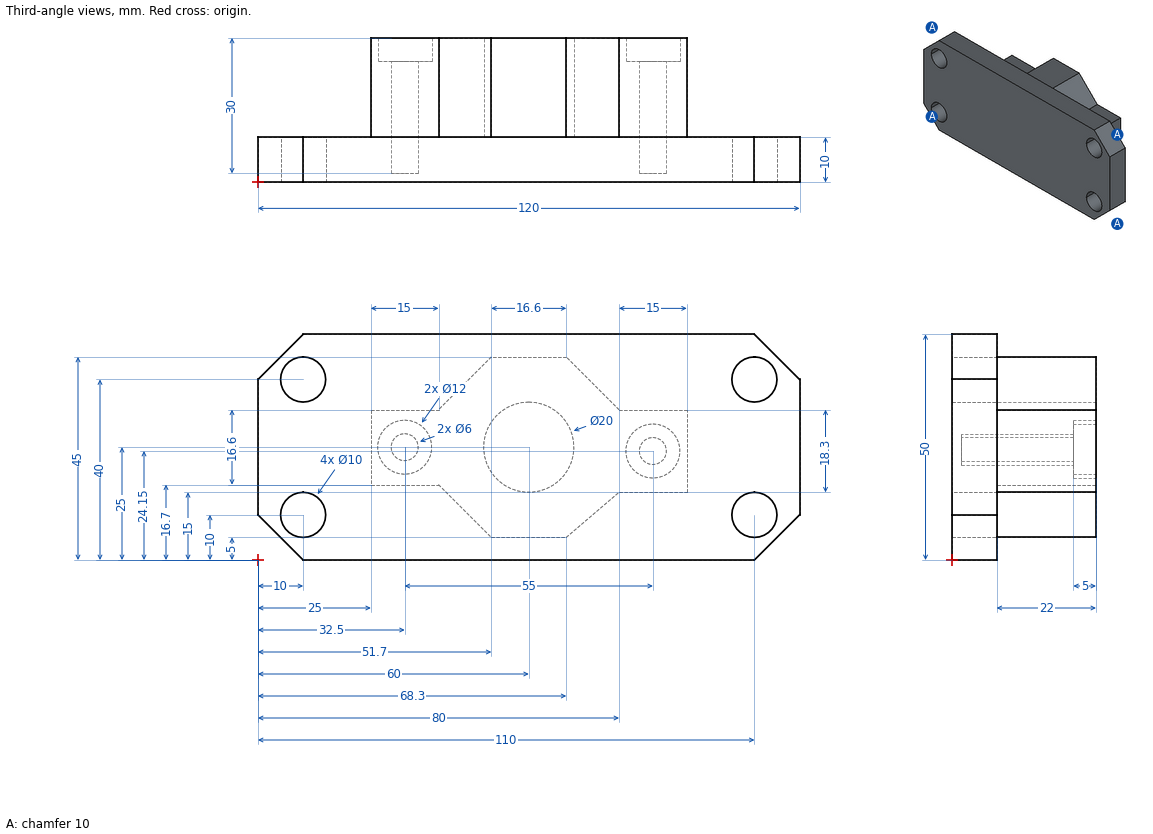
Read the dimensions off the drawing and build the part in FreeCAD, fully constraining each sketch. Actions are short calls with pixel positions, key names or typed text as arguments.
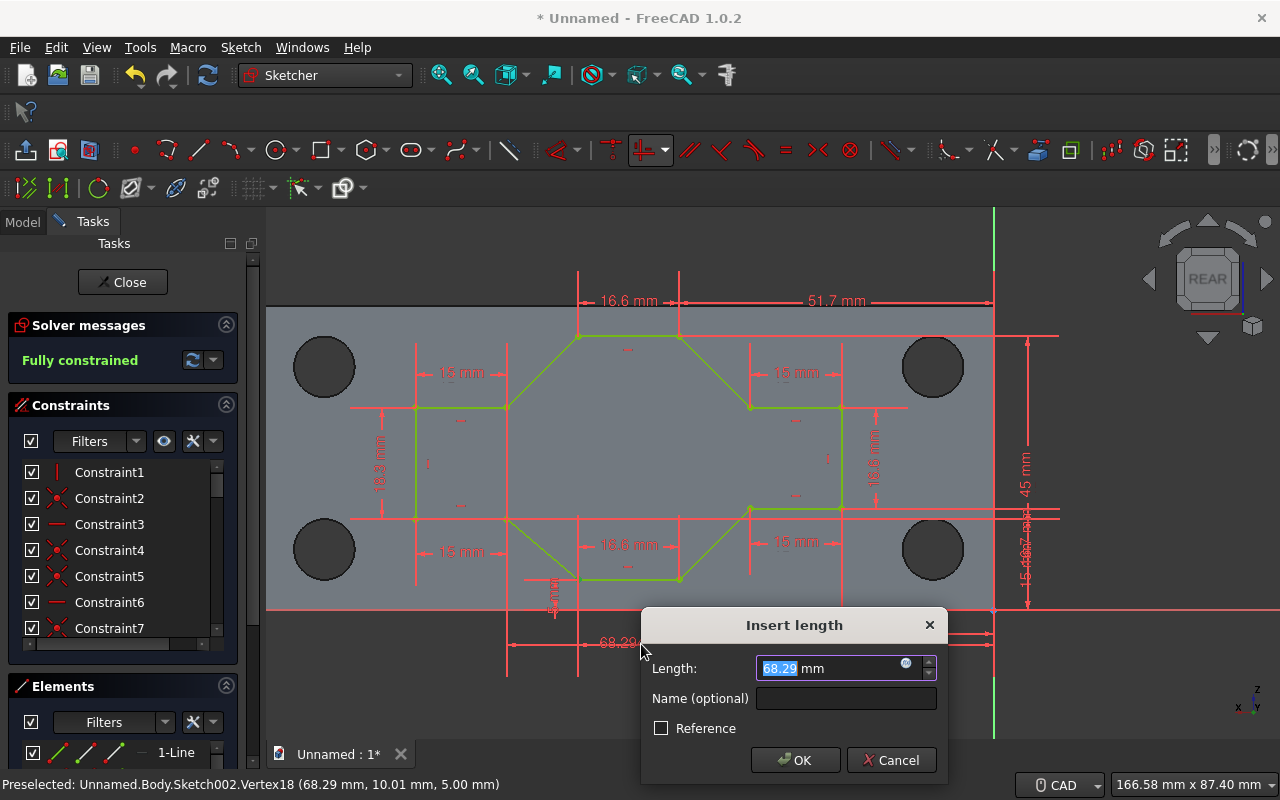
text(68.3)
key(Return)
key(Escape)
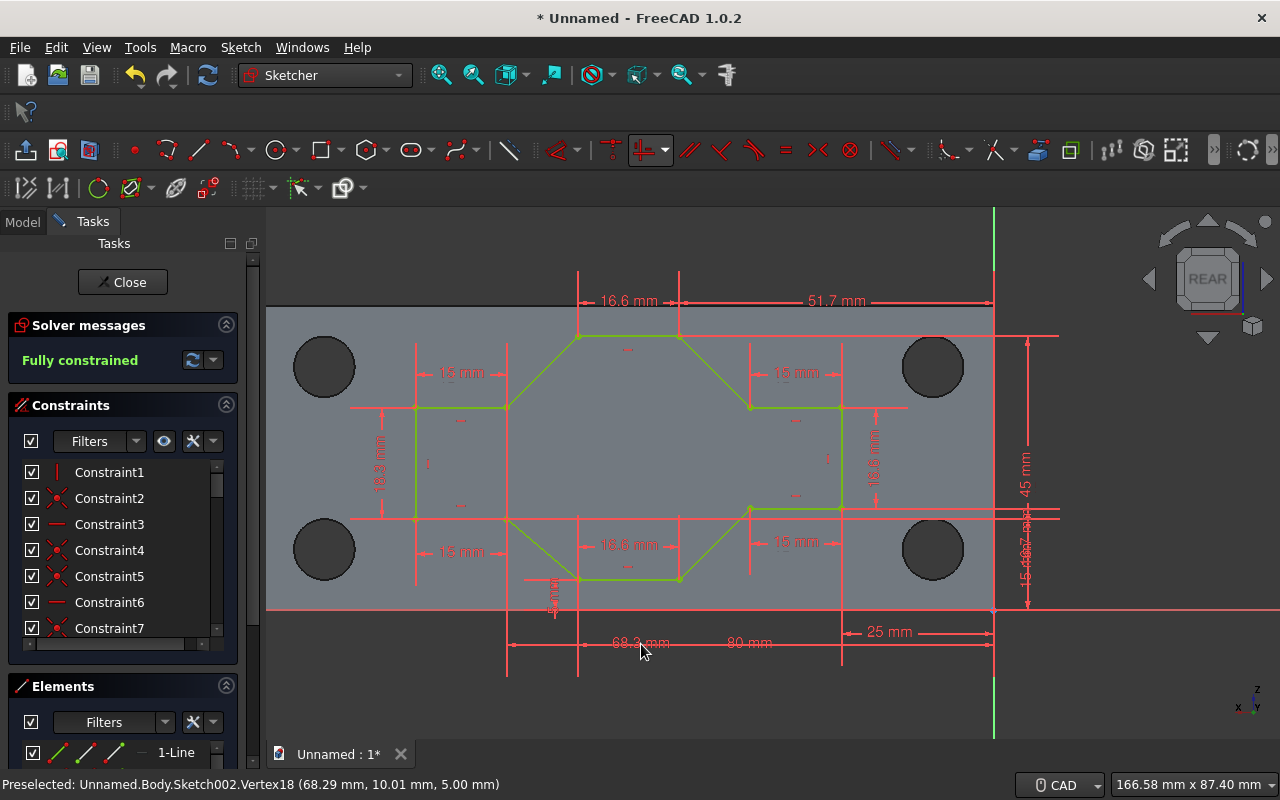
click(123, 282)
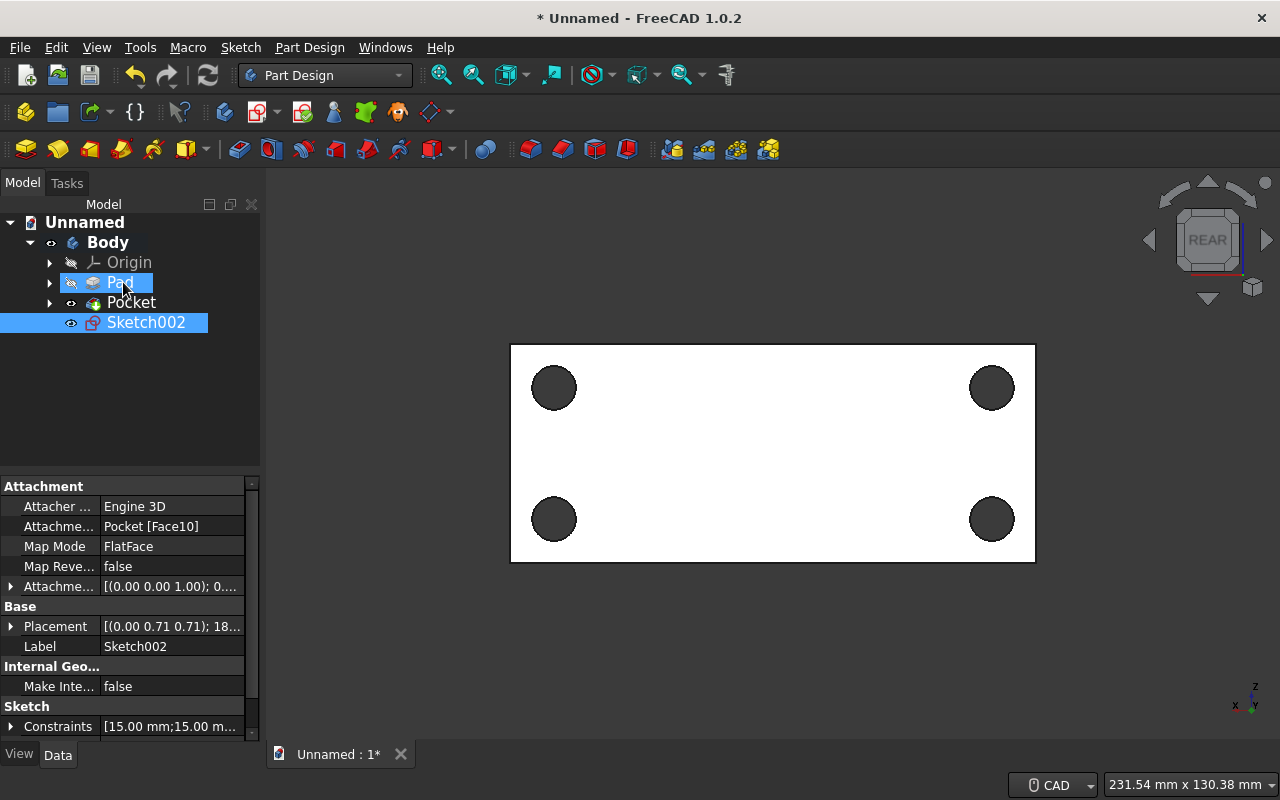
click(26, 150)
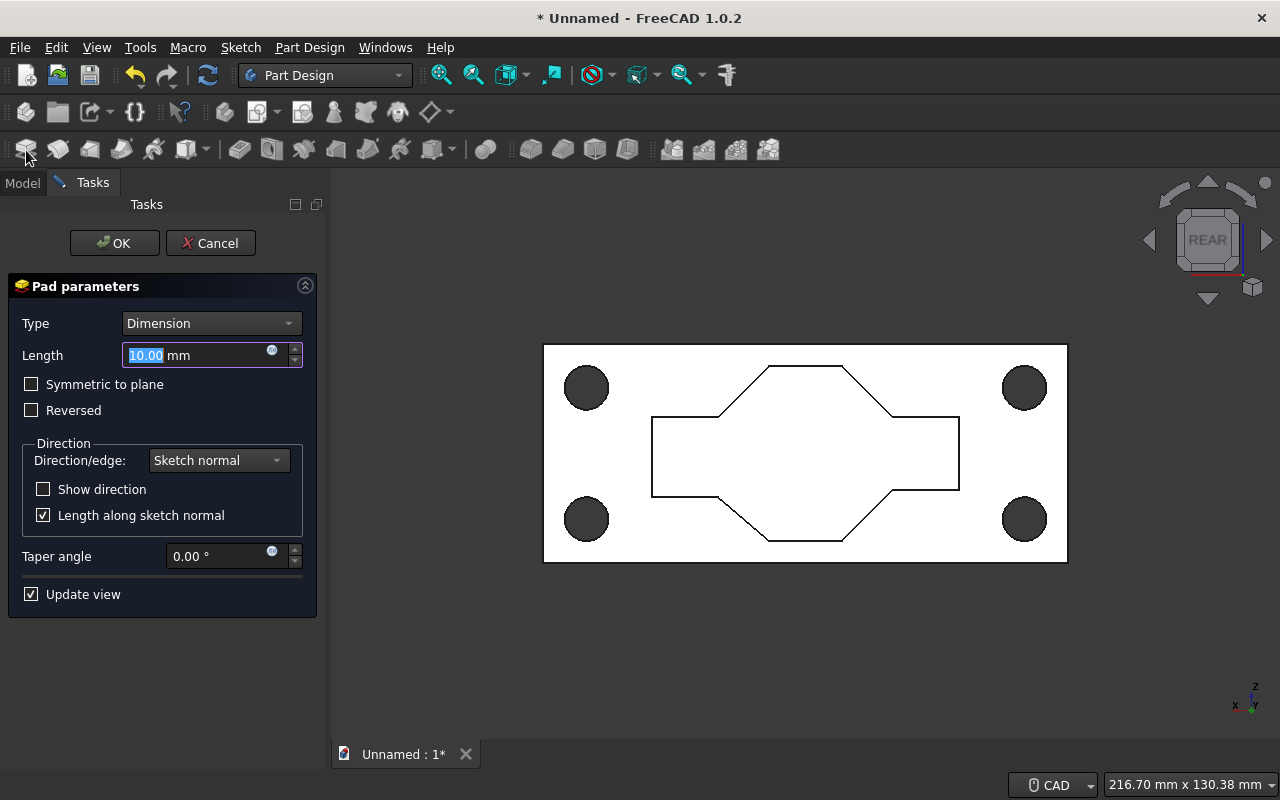
text(22)
key(Tab)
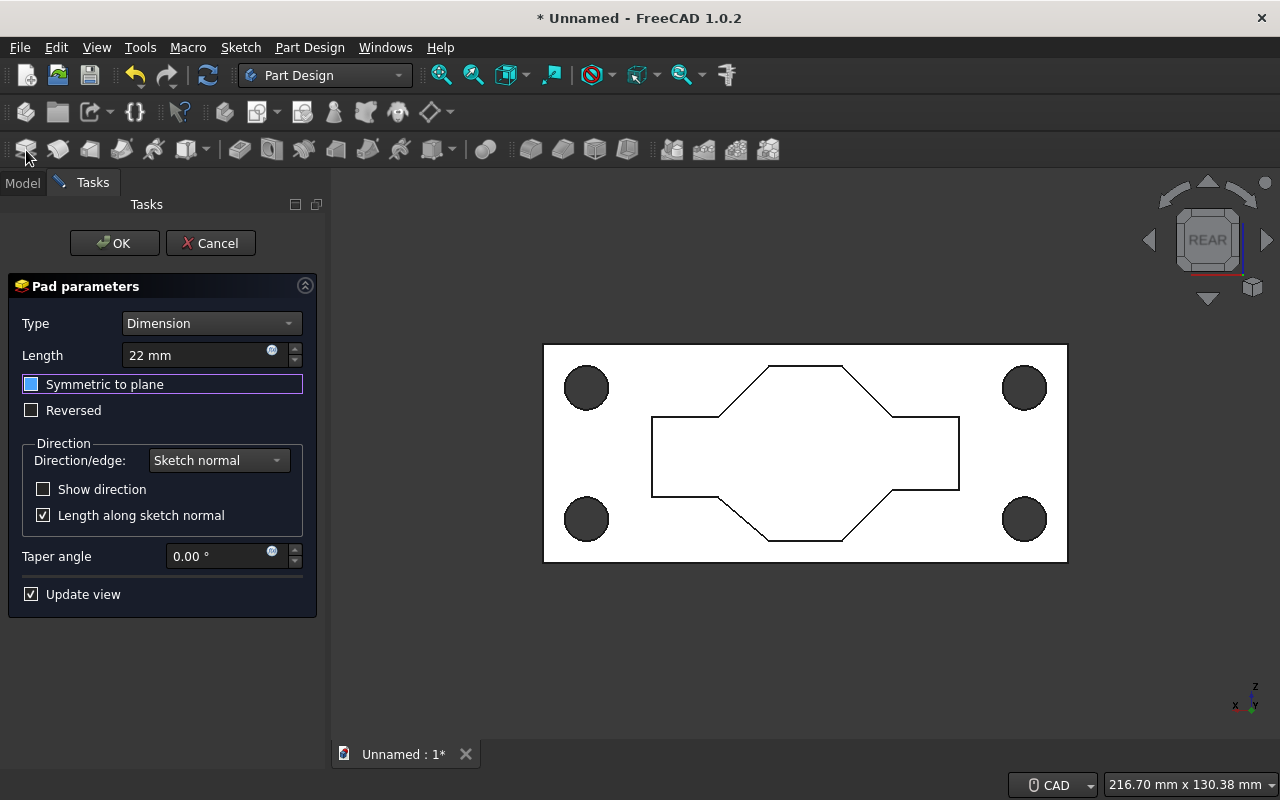
click(115, 243)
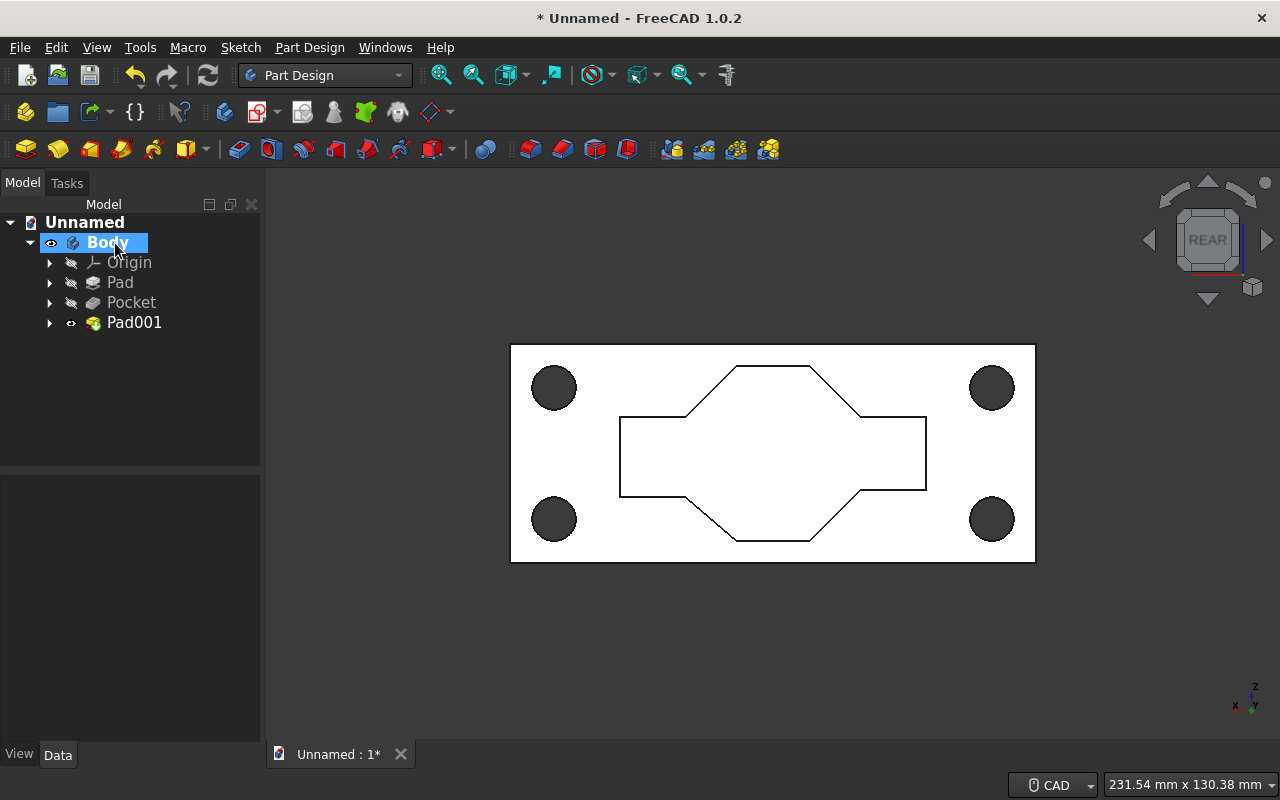
click(773, 452)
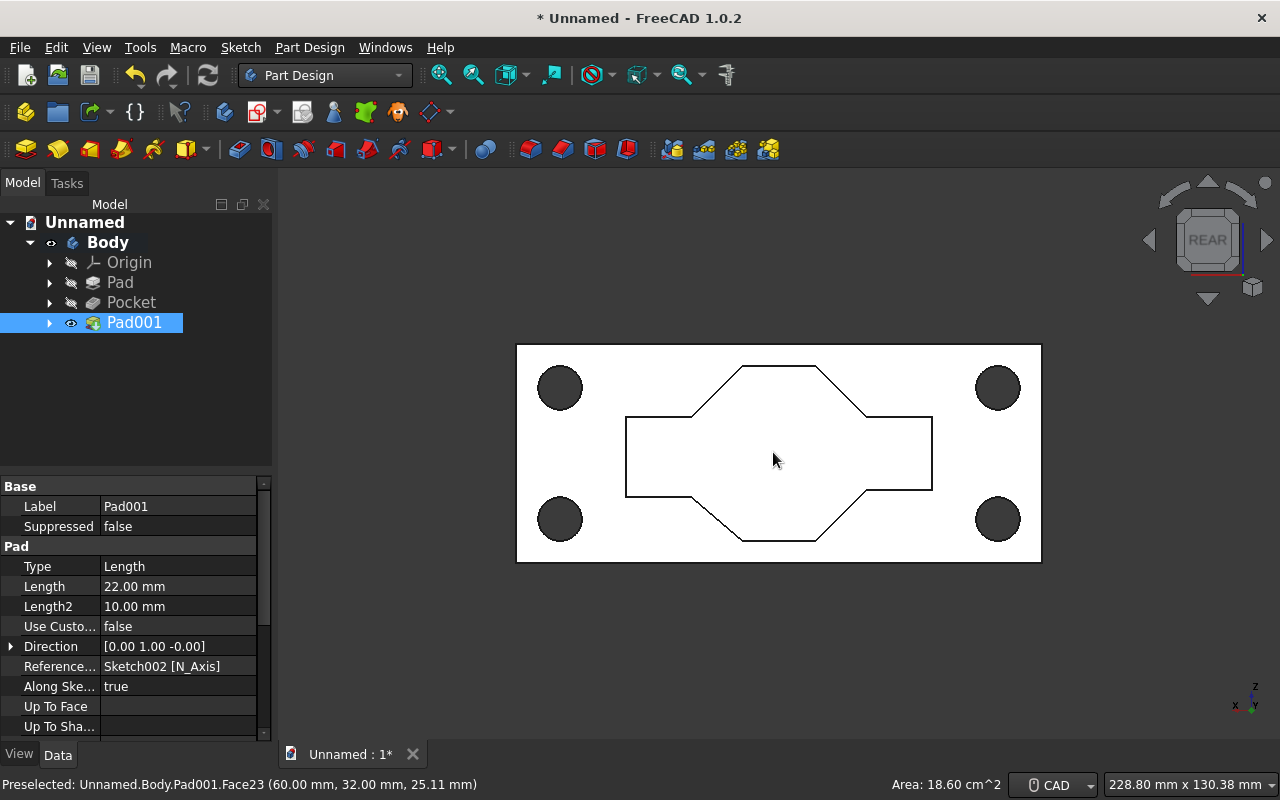
click(258, 112)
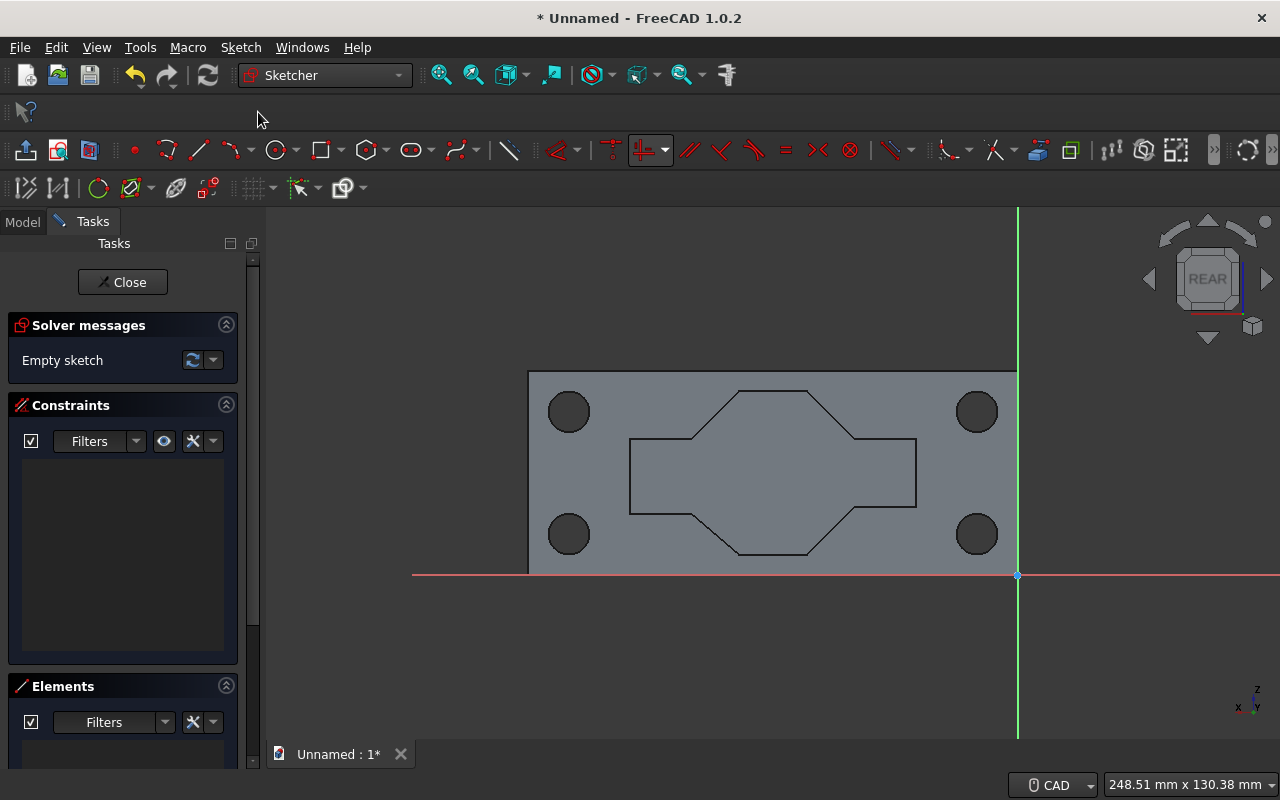
scroll(795, 473, up, 7)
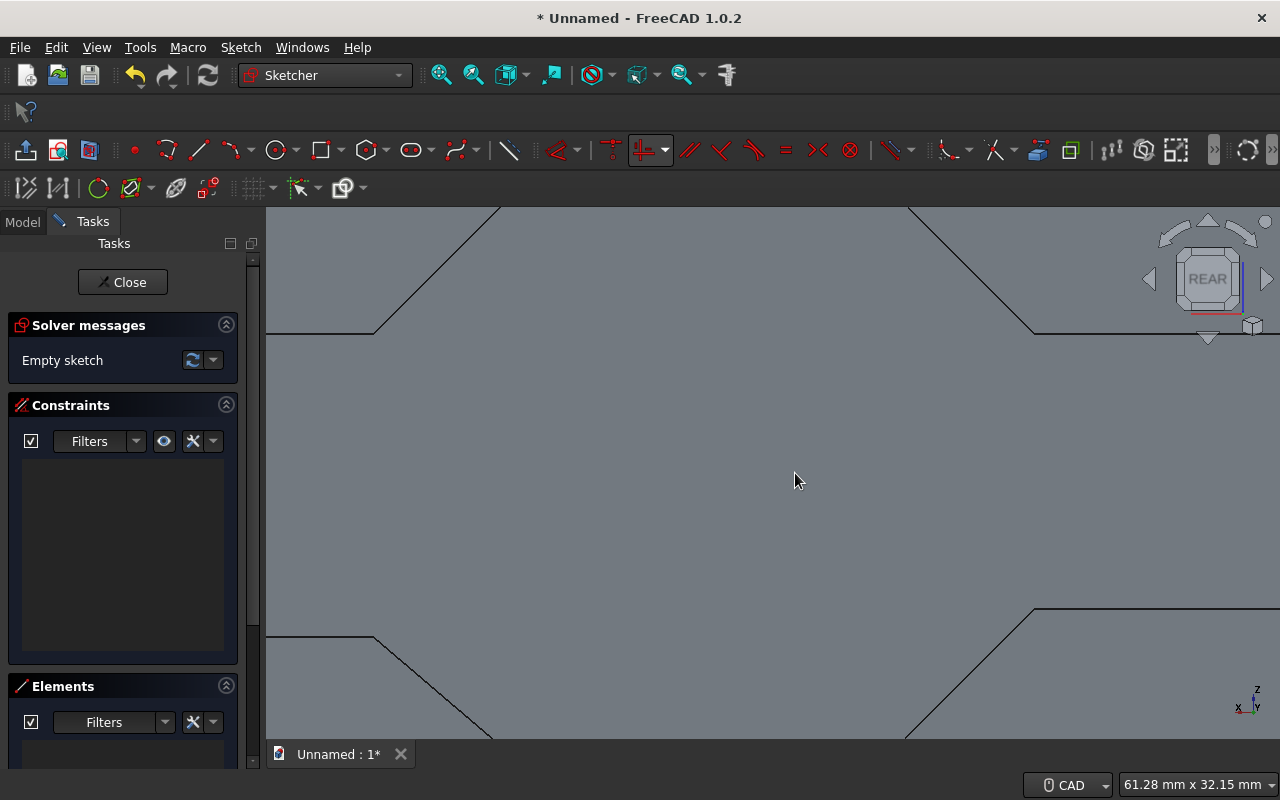
click(276, 150)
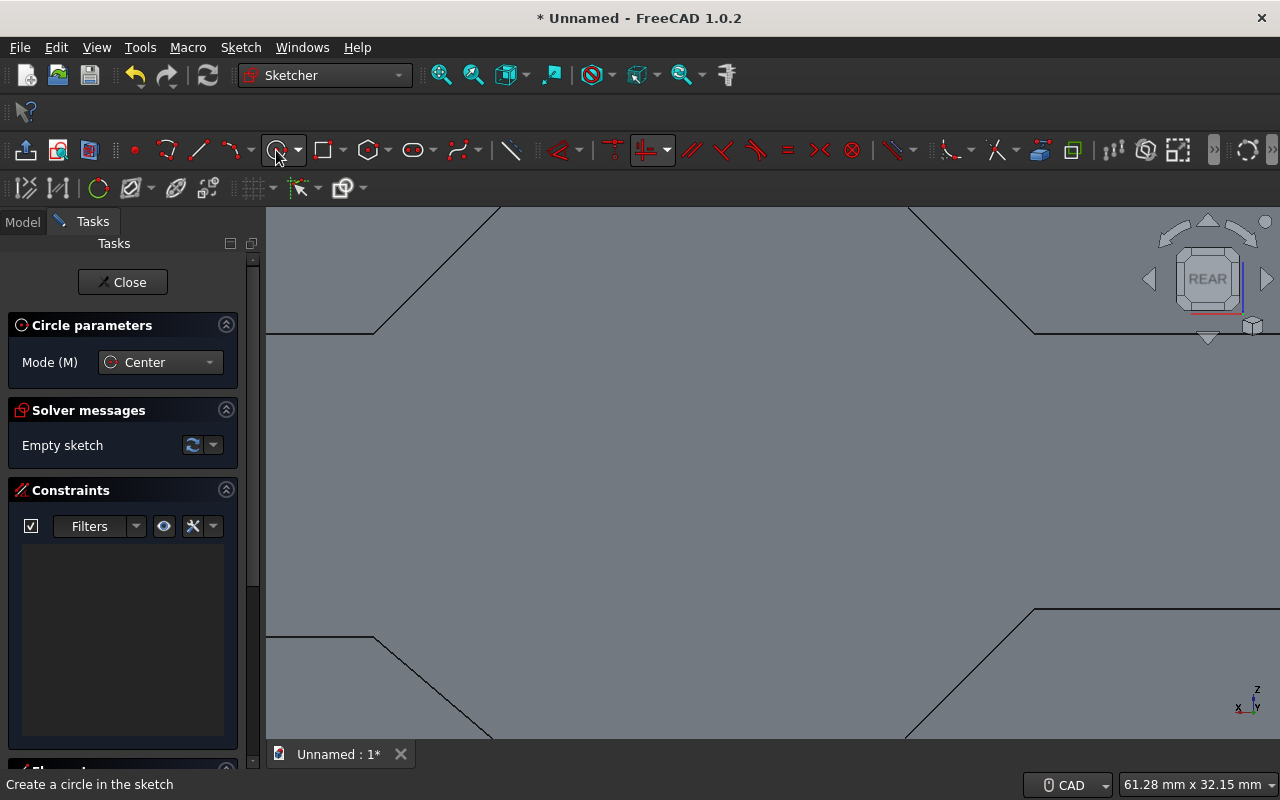
click(704, 471)
click(821, 354)
key(Escape)